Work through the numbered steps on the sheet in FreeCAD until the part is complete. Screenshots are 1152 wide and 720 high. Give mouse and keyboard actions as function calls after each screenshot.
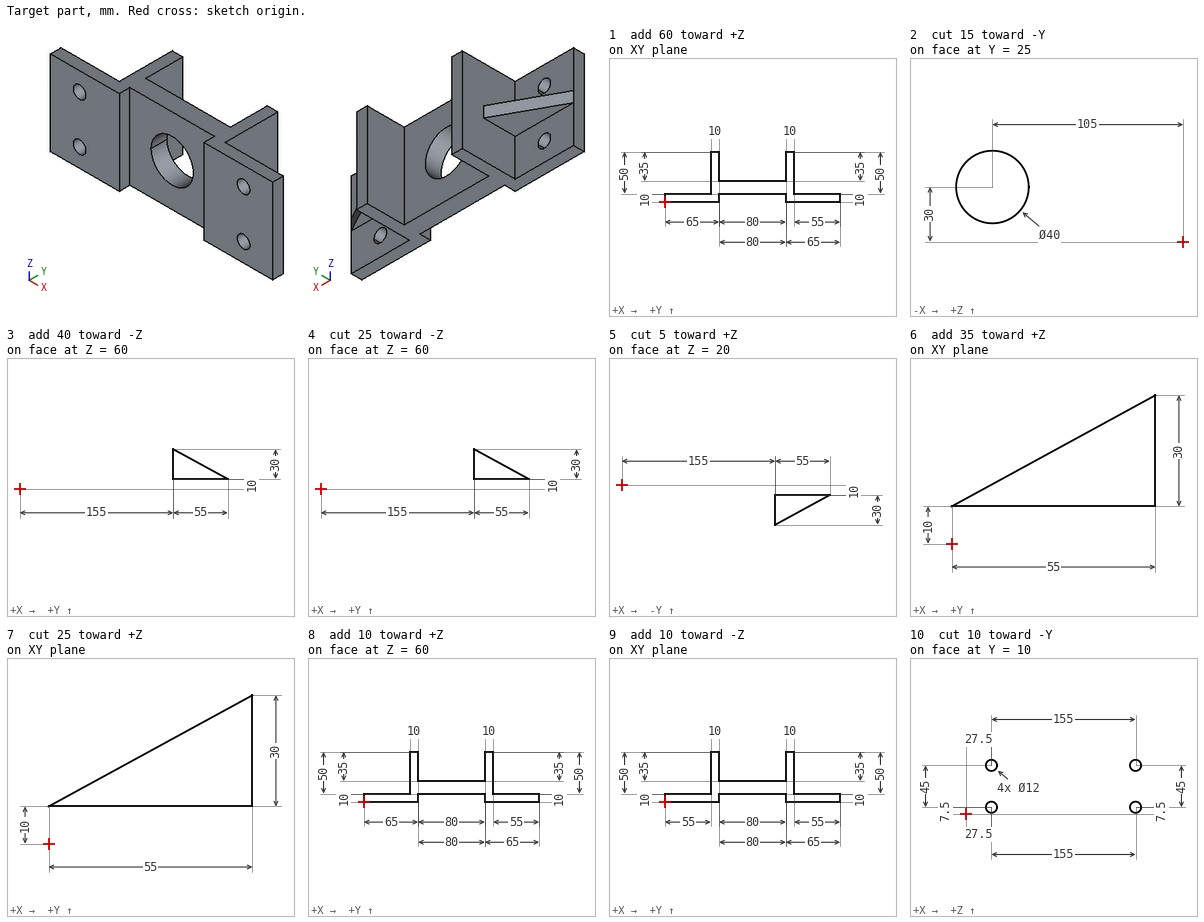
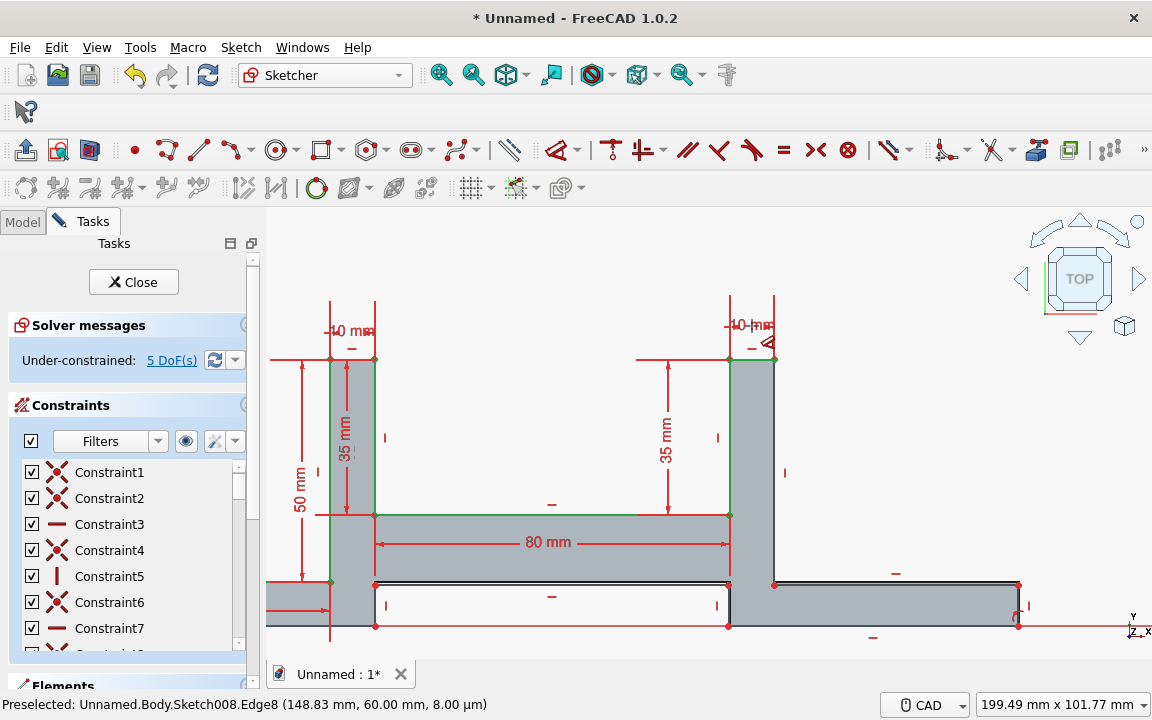
click(774, 428)
click(808, 473)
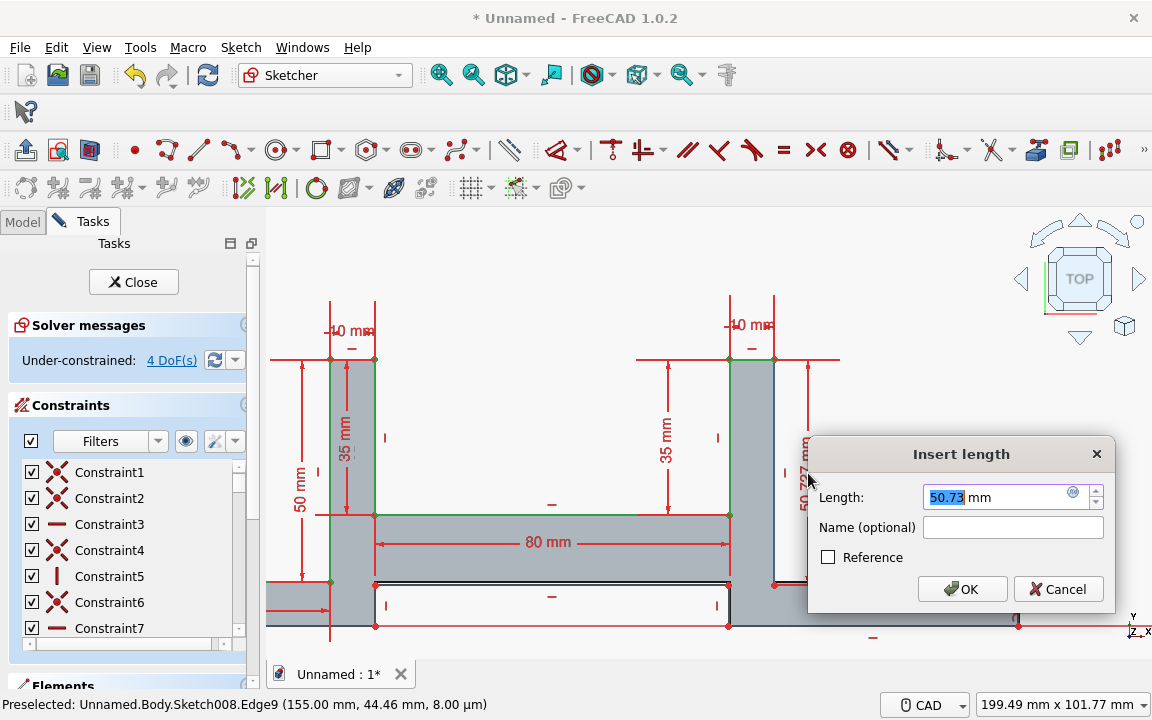
text(50)
key(Return)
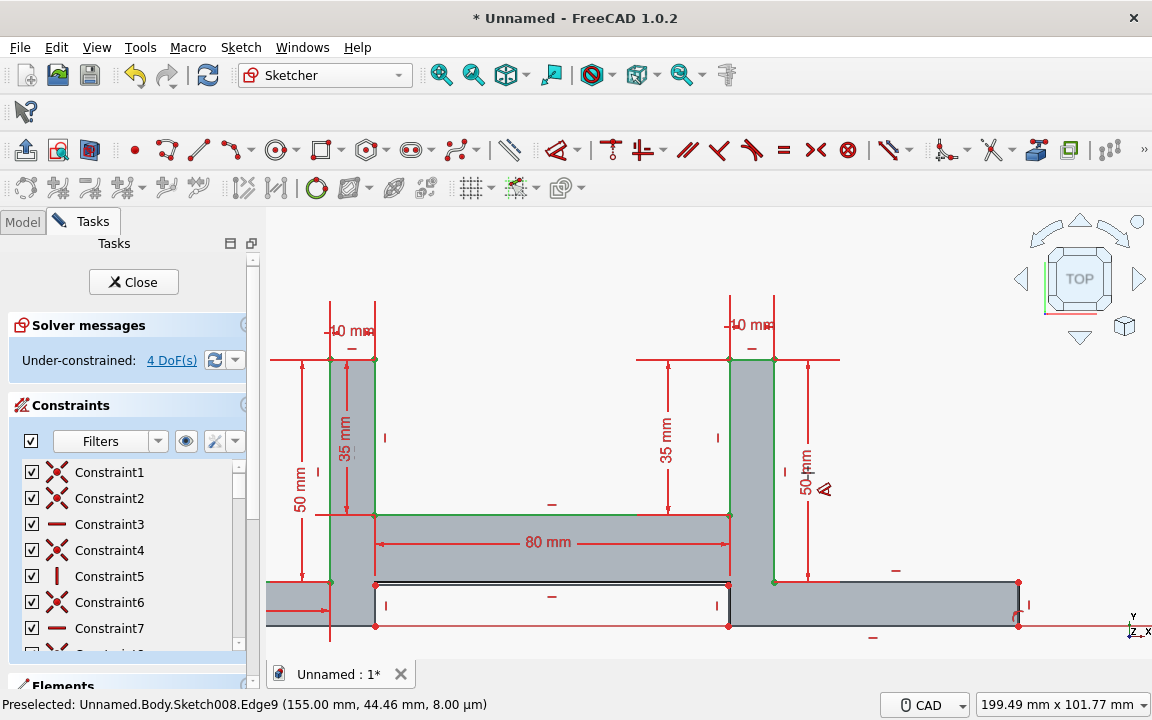
click(848, 582)
click(881, 548)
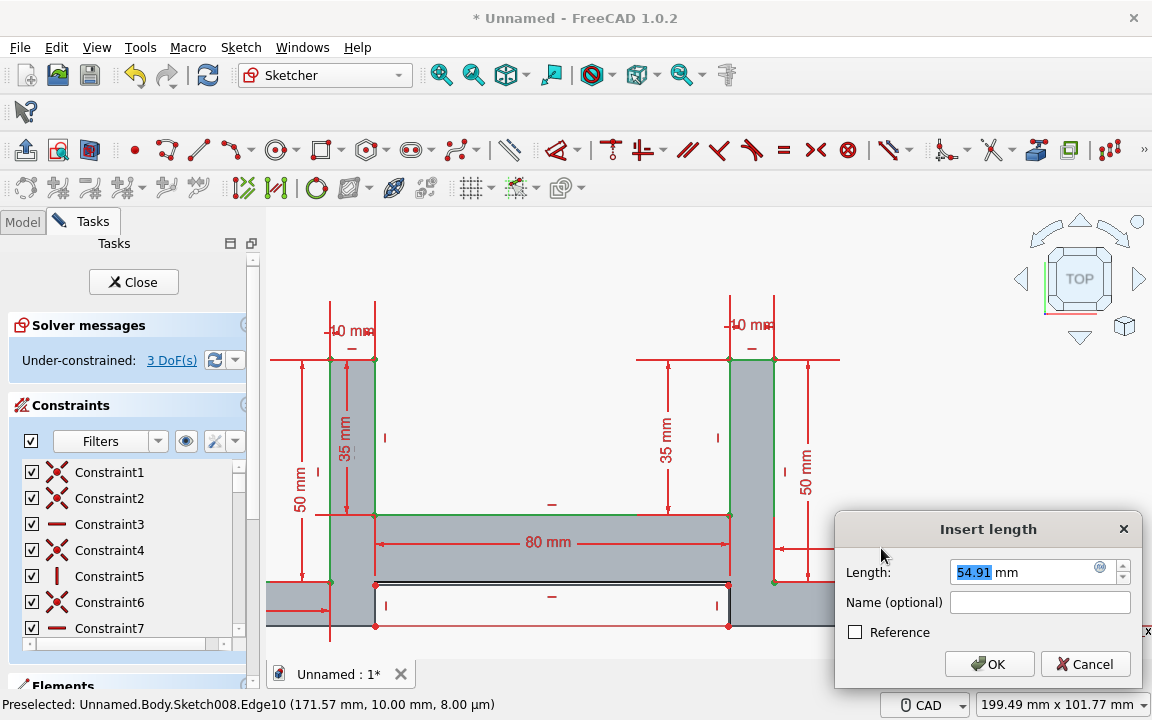
text(55)
key(Return)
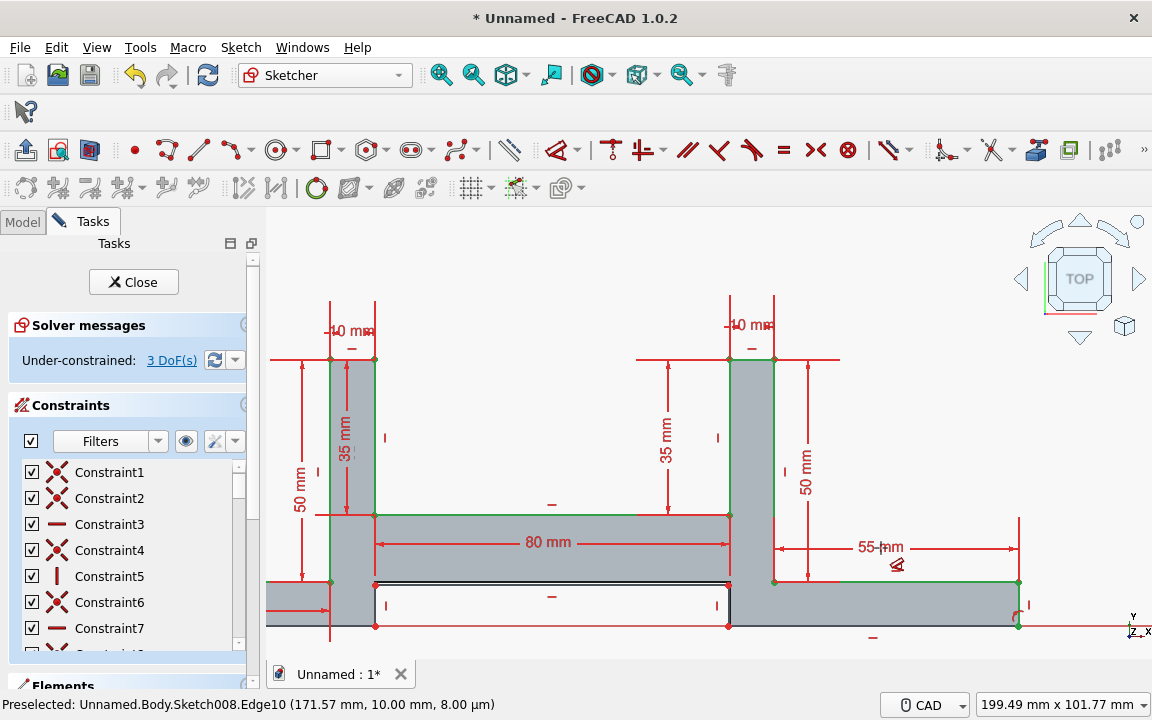
click(932, 626)
click(858, 568)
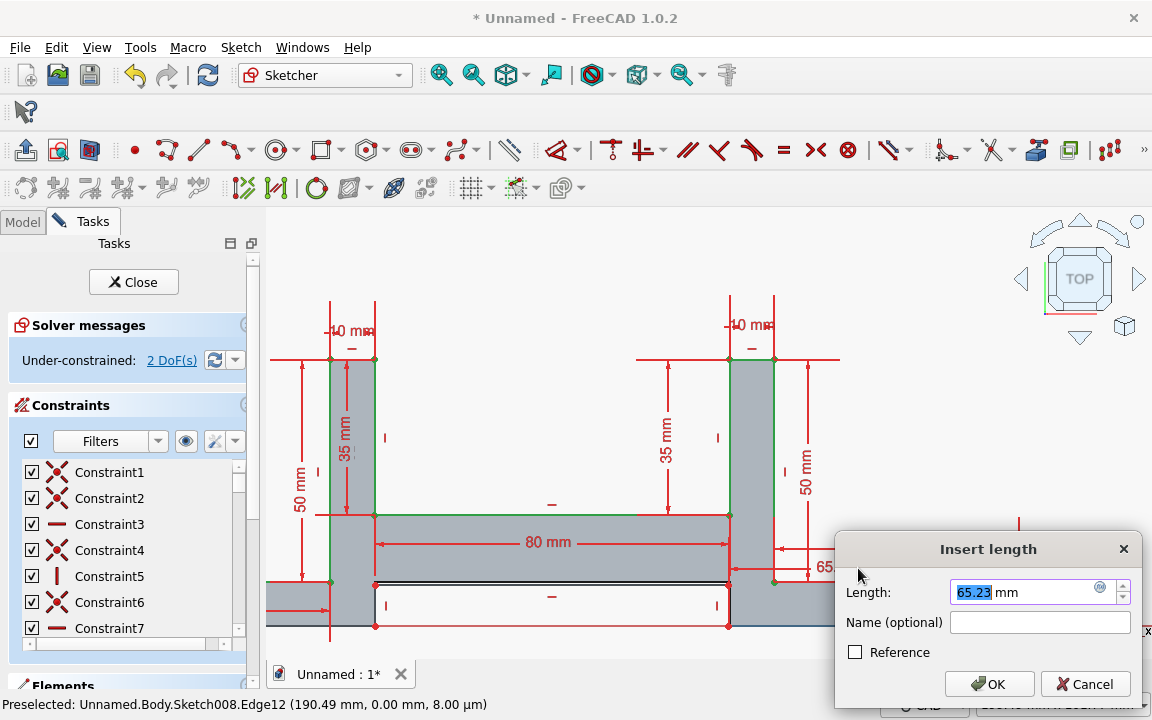
text(65)
key(Return)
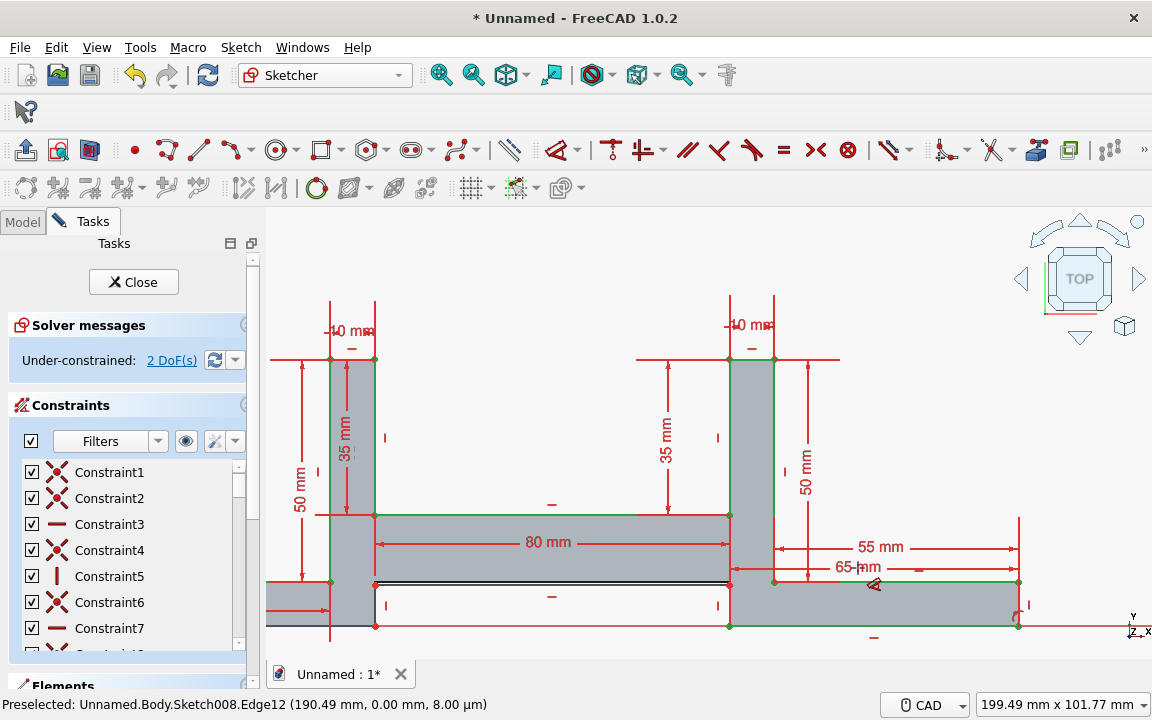
click(730, 614)
click(764, 606)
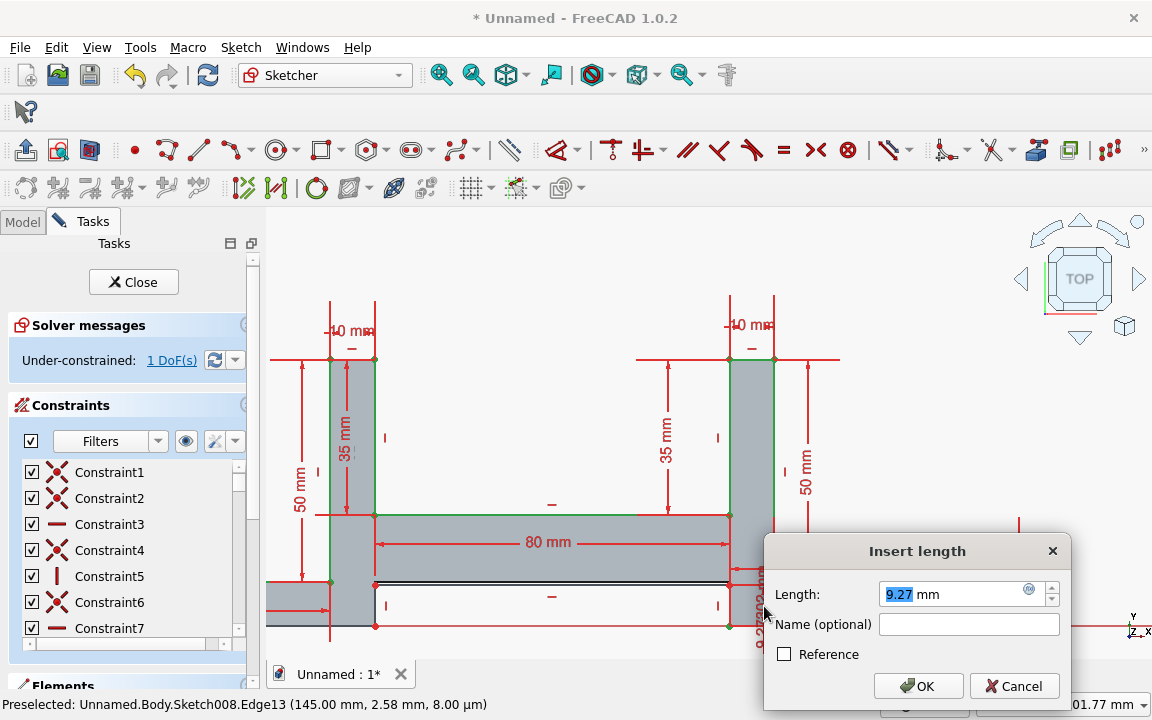
text(10)
key(Return)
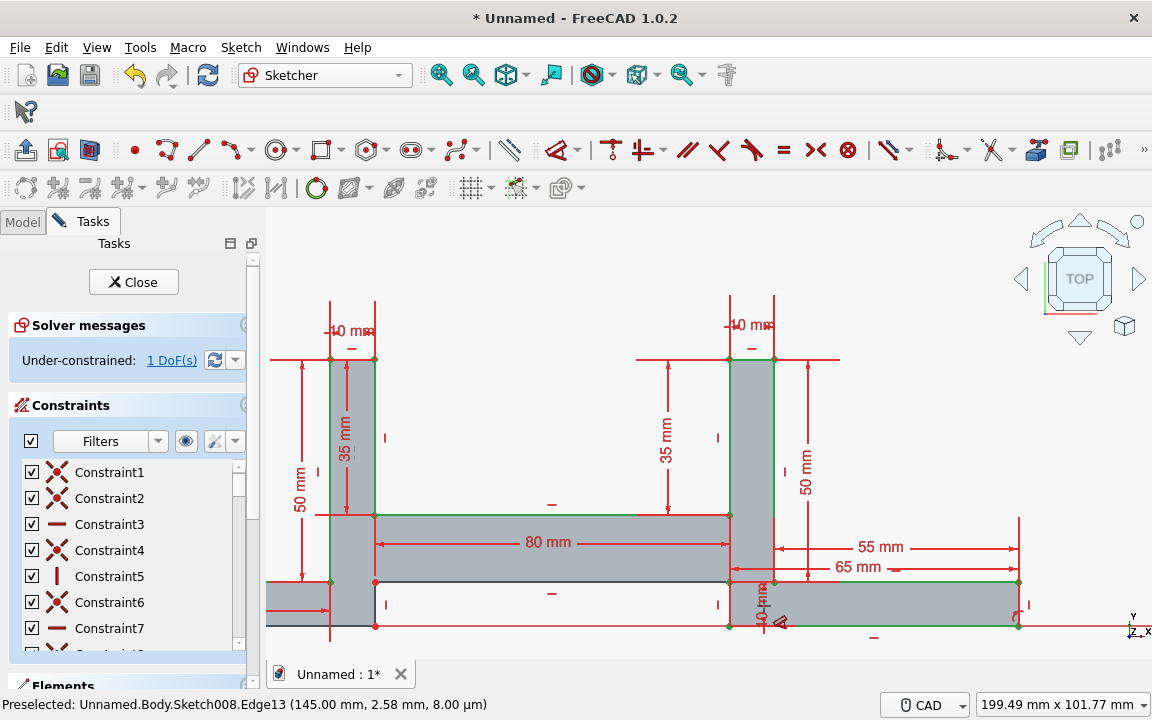
click(624, 582)
click(471, 548)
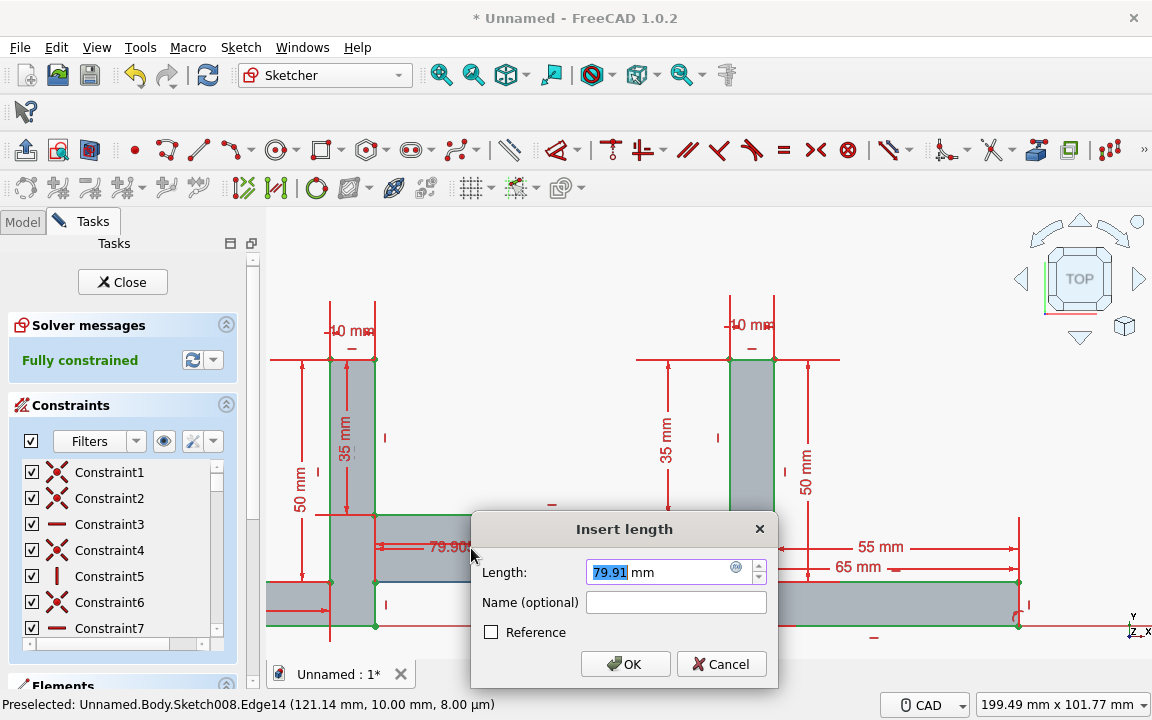
text(80)
key(Return)
key(Escape)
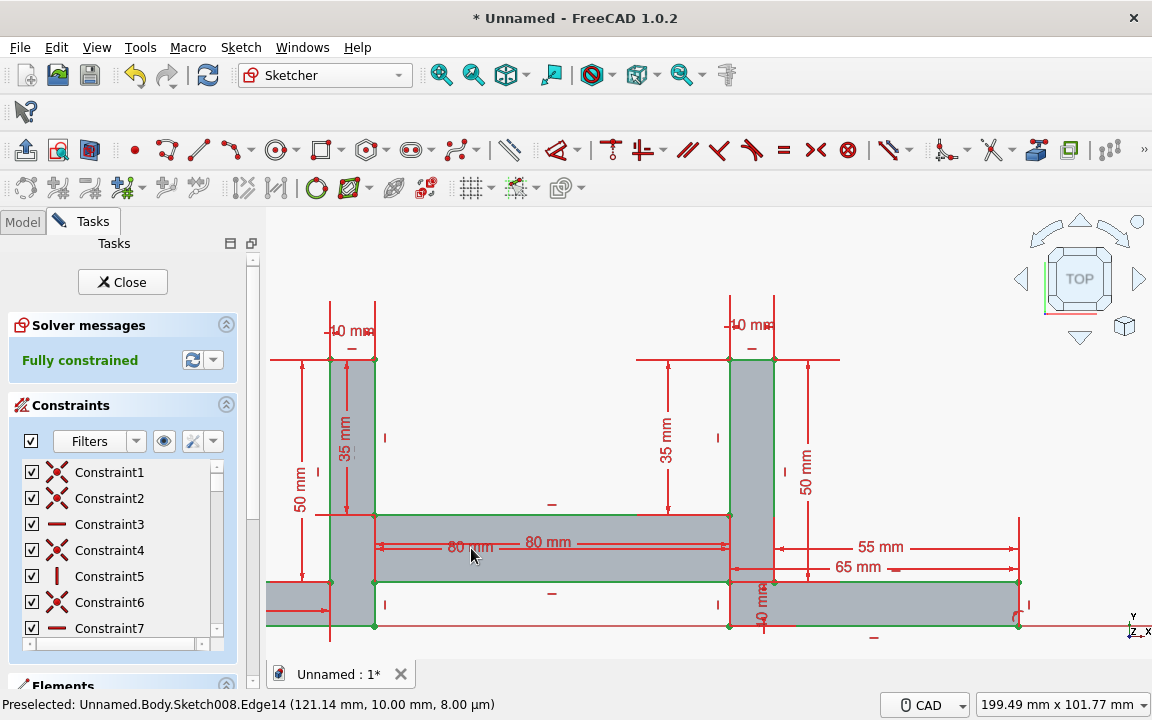
click(123, 282)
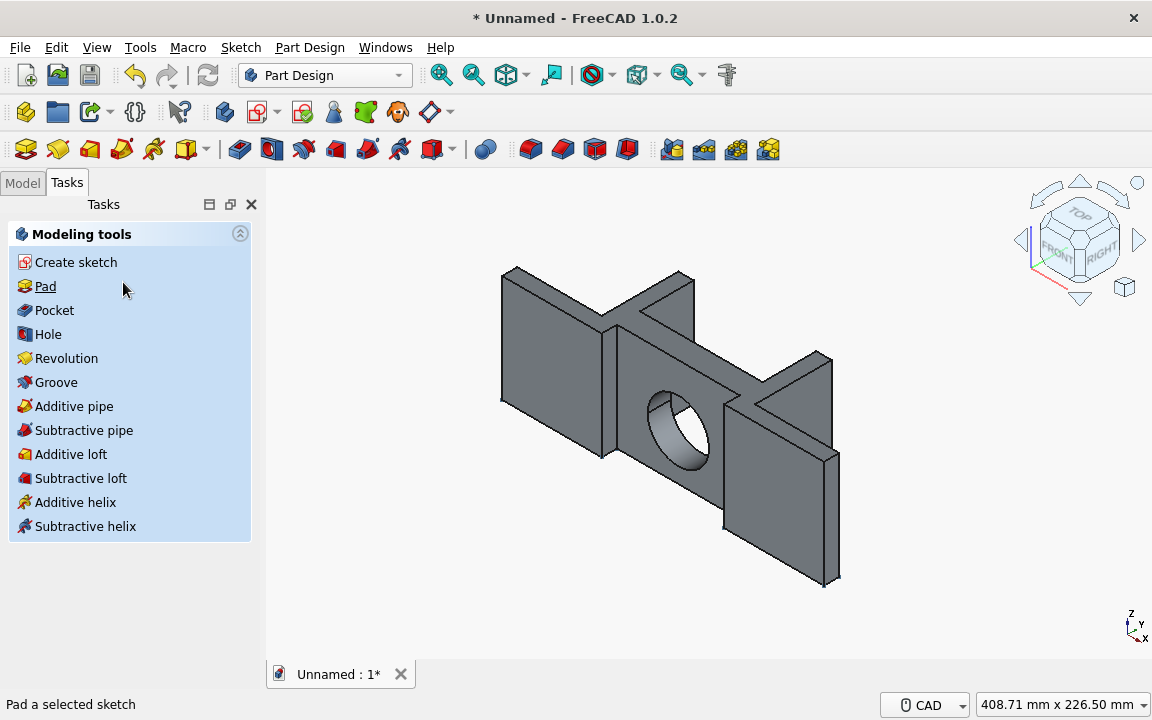
click(26, 150)